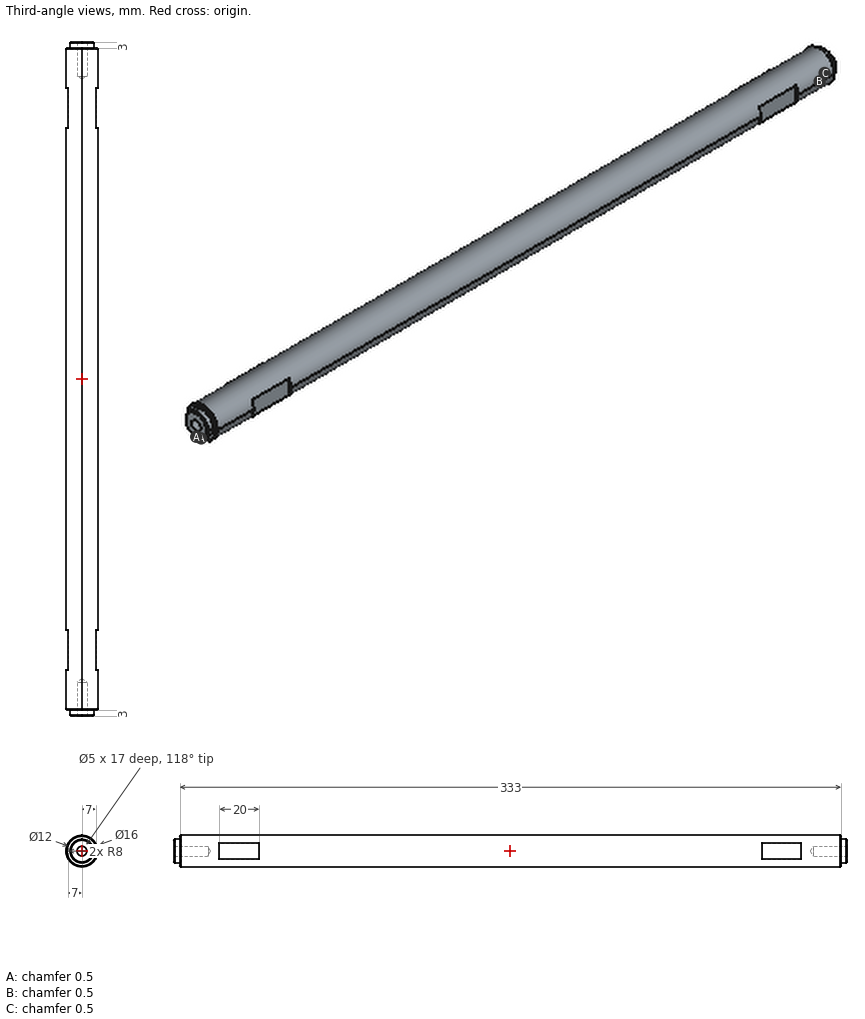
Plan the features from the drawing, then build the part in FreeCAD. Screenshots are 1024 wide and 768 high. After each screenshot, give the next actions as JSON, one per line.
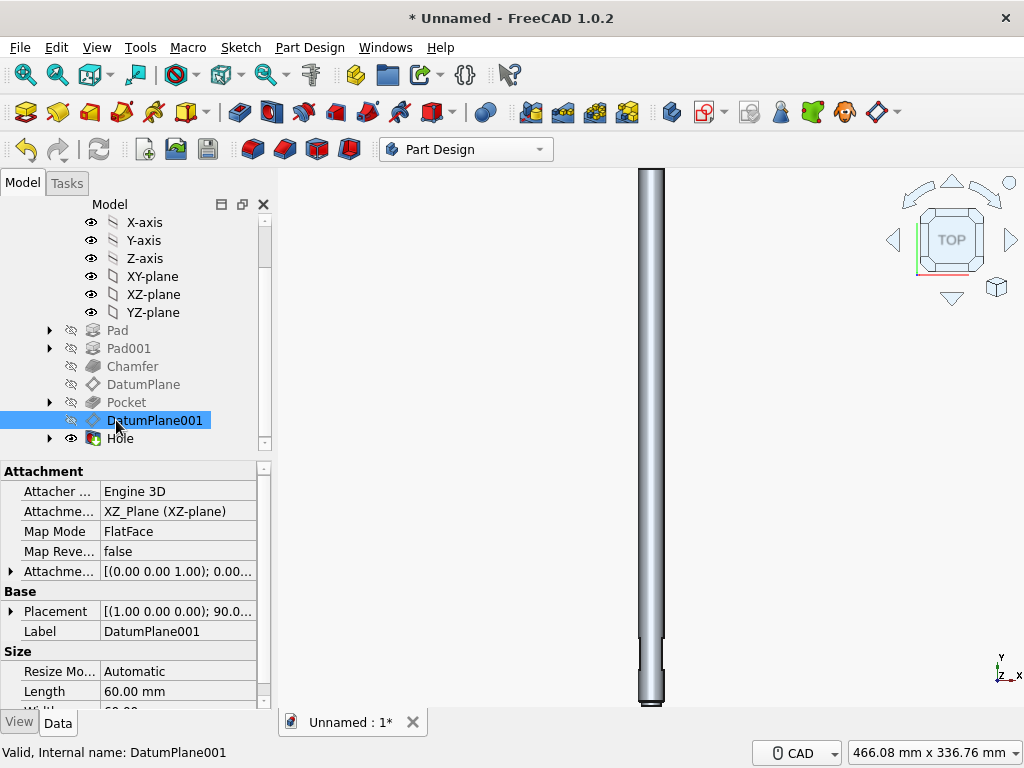
{"action": "key", "text": "0"}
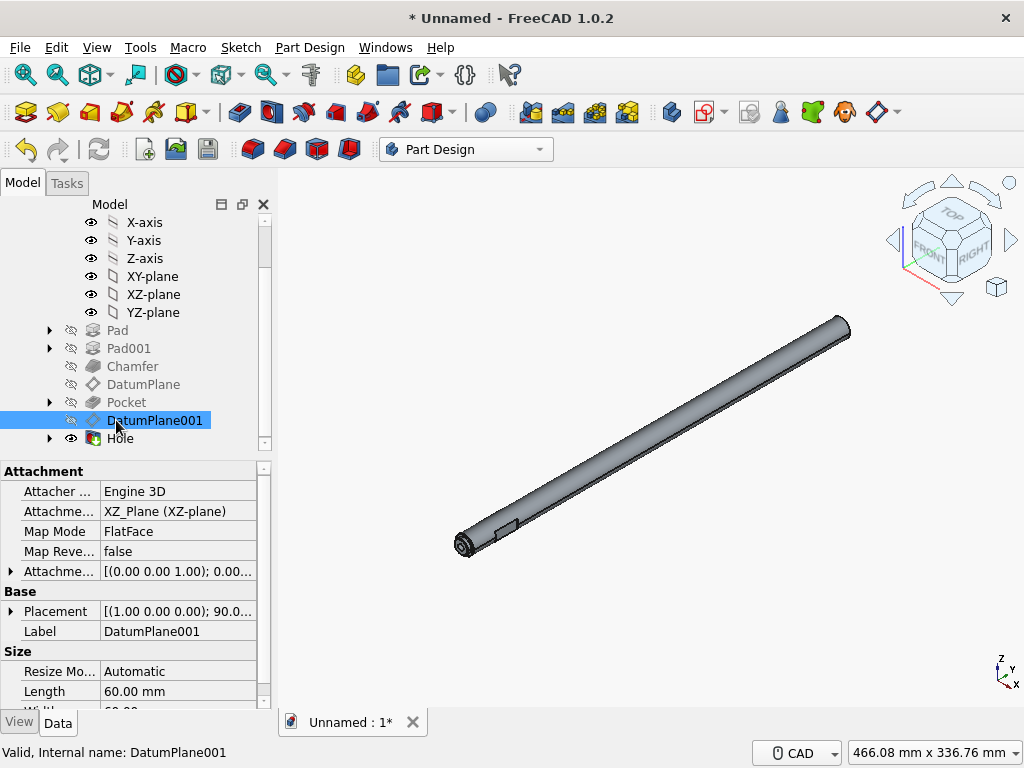
{"action": "left_click", "coordinate": [838, 315]}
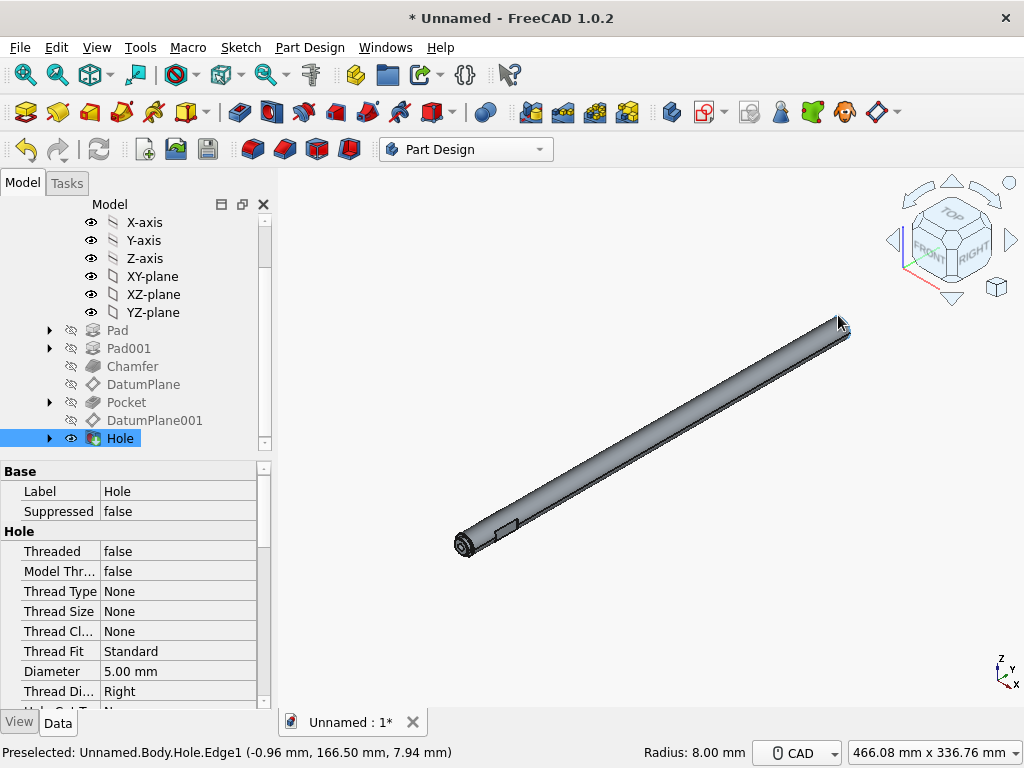
{"action": "left_click", "coordinate": [286, 150]}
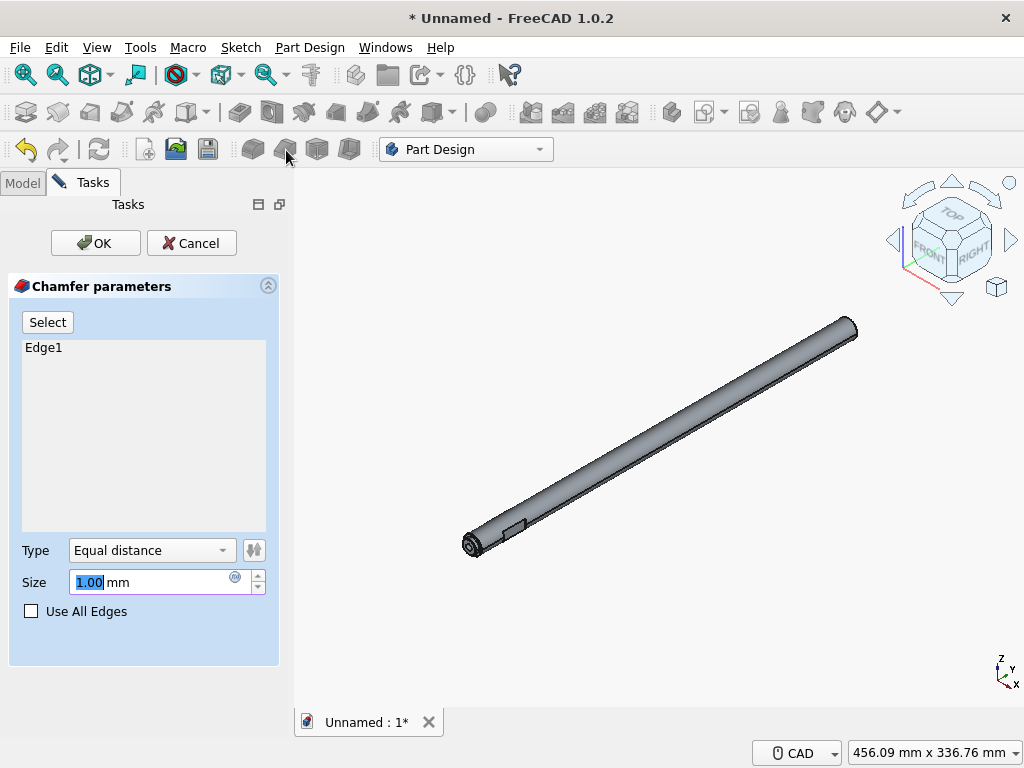
{"action": "type", "text": "0.5"}
{"action": "key", "text": "Tab"}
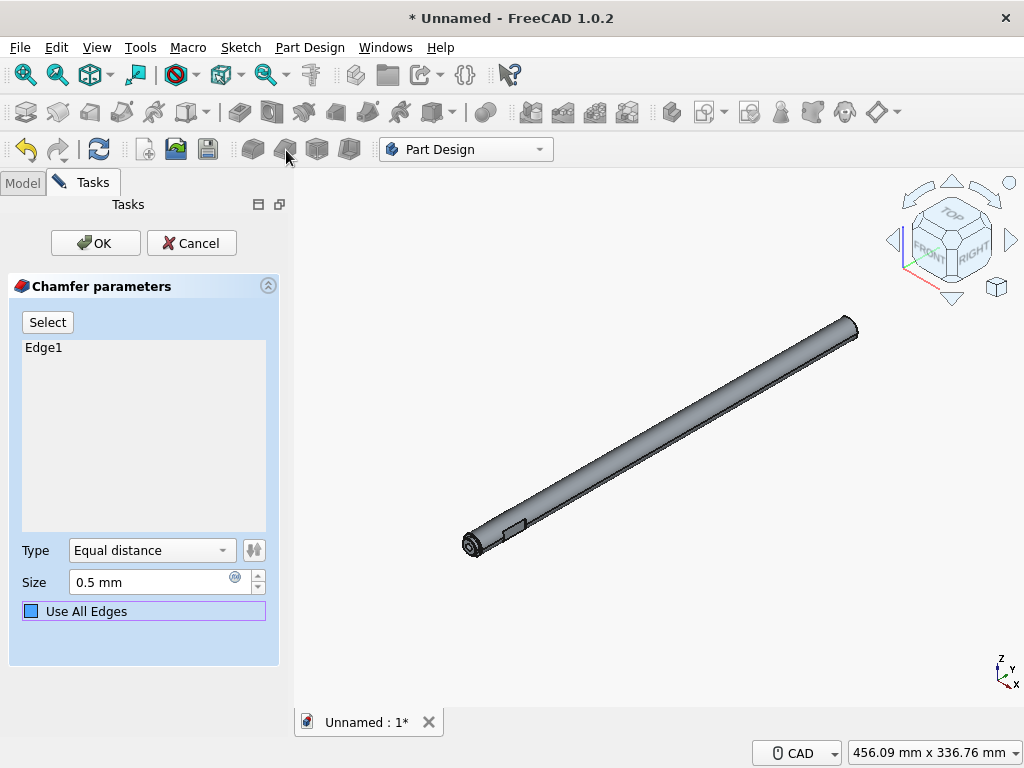
{"action": "left_click", "coordinate": [96, 243]}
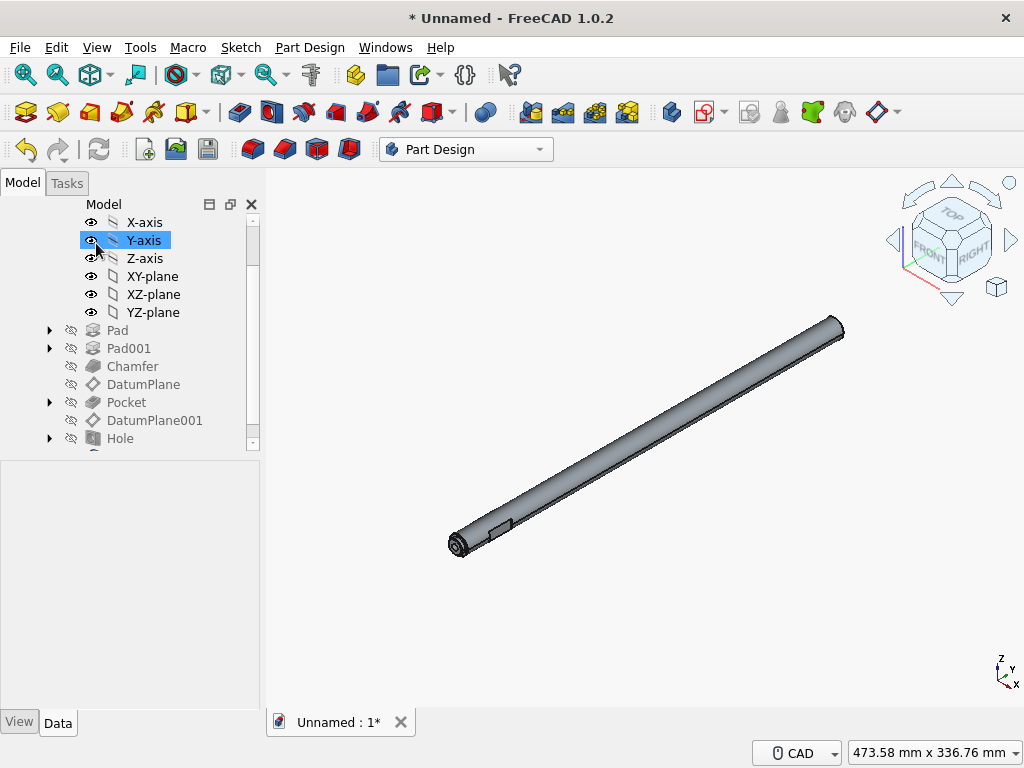
{"action": "scroll", "coordinate": [160, 326], "scroll_direction": "down", "scroll_amount": 3}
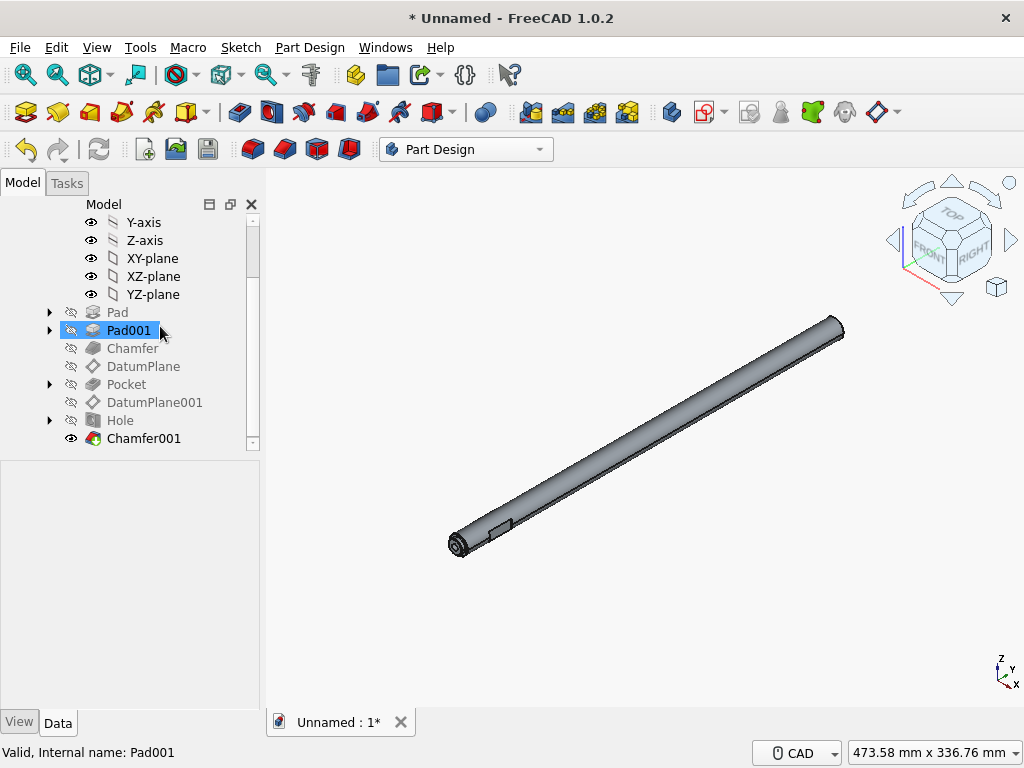
{"action": "scroll", "coordinate": [160, 326], "scroll_direction": "up", "scroll_amount": 15}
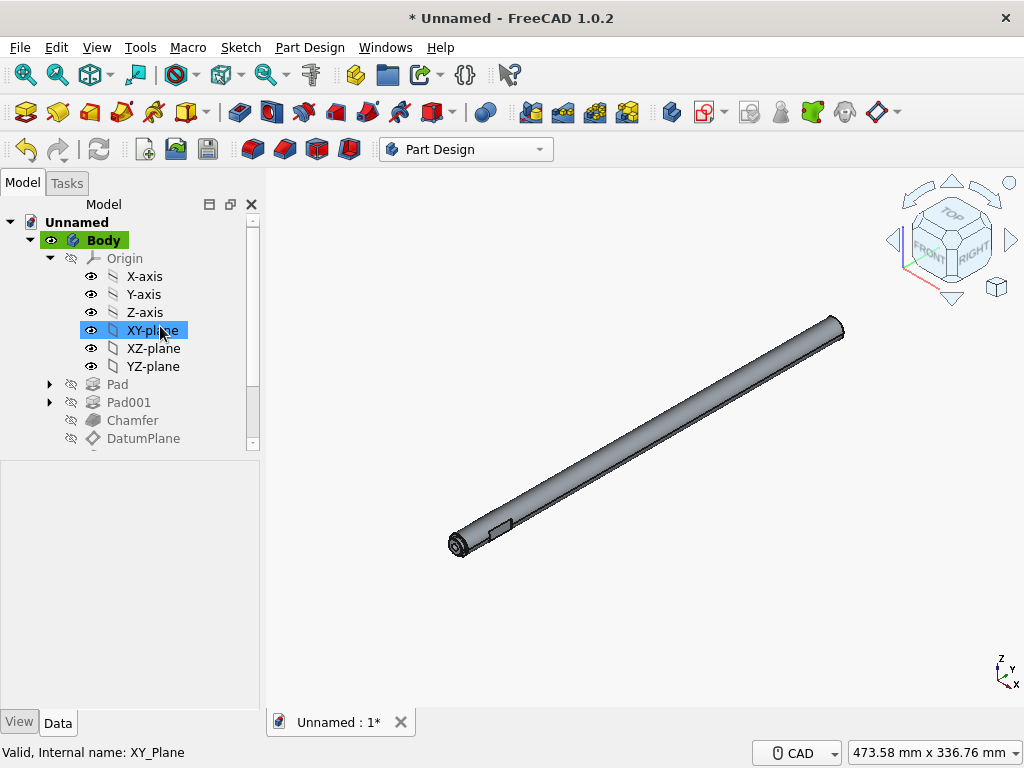
{"action": "left_click", "coordinate": [136, 348]}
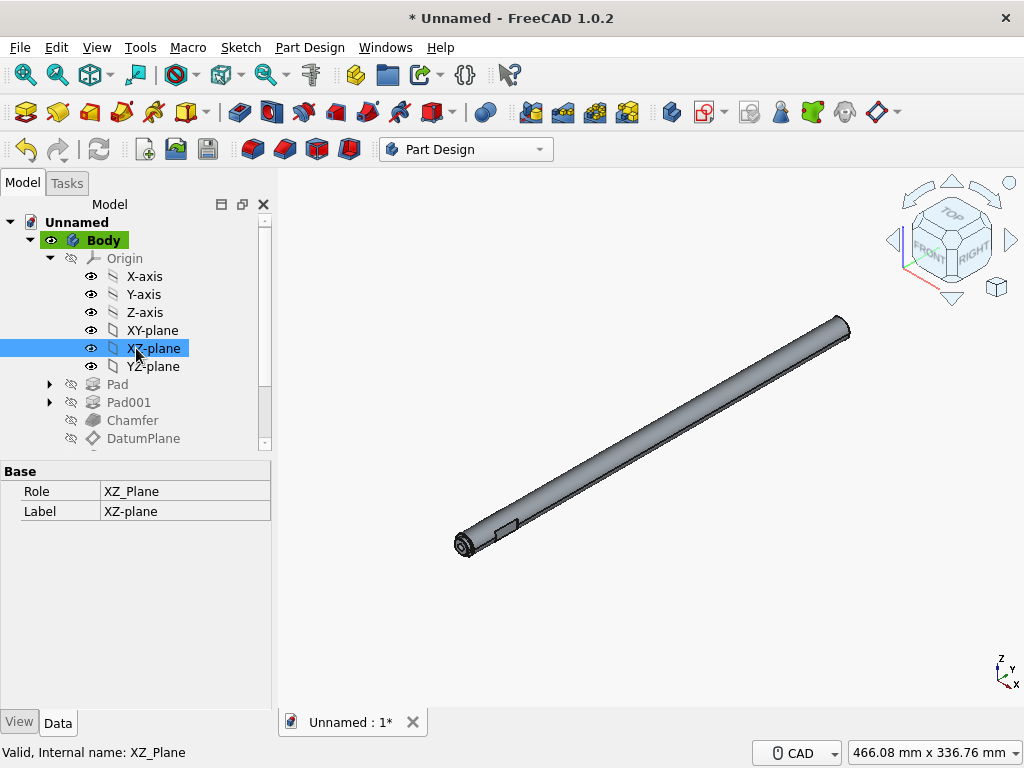
{"action": "left_click", "coordinate": [878, 112]}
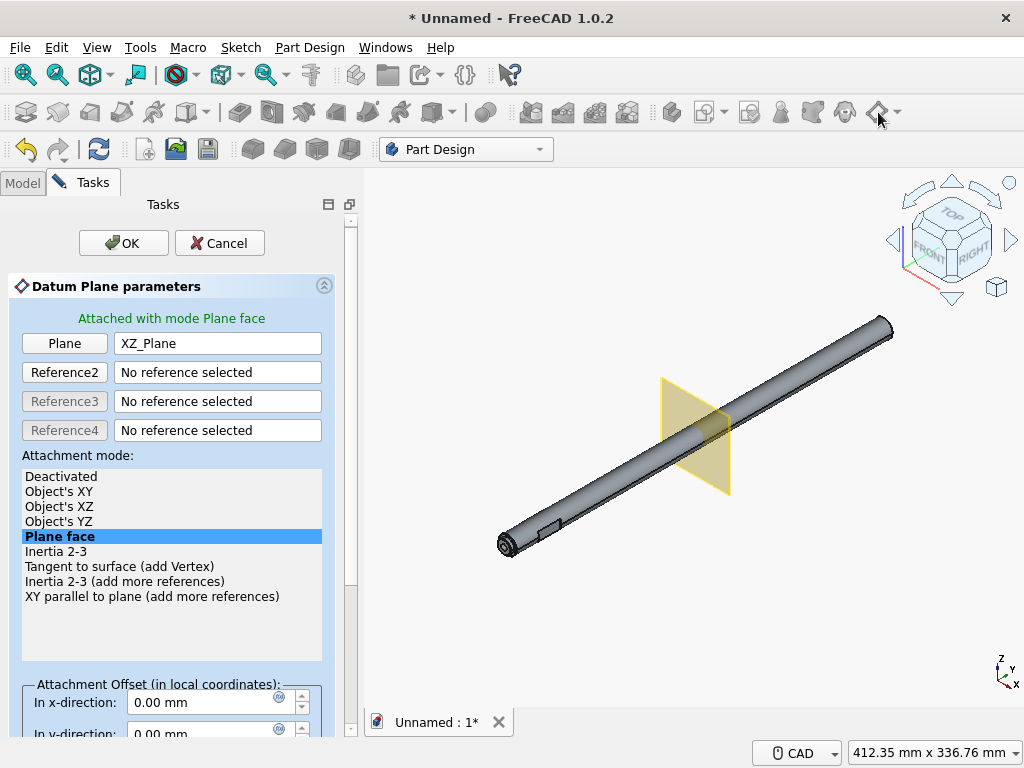
{"action": "scroll", "coordinate": [351, 475], "scroll_direction": "down", "scroll_amount": 2}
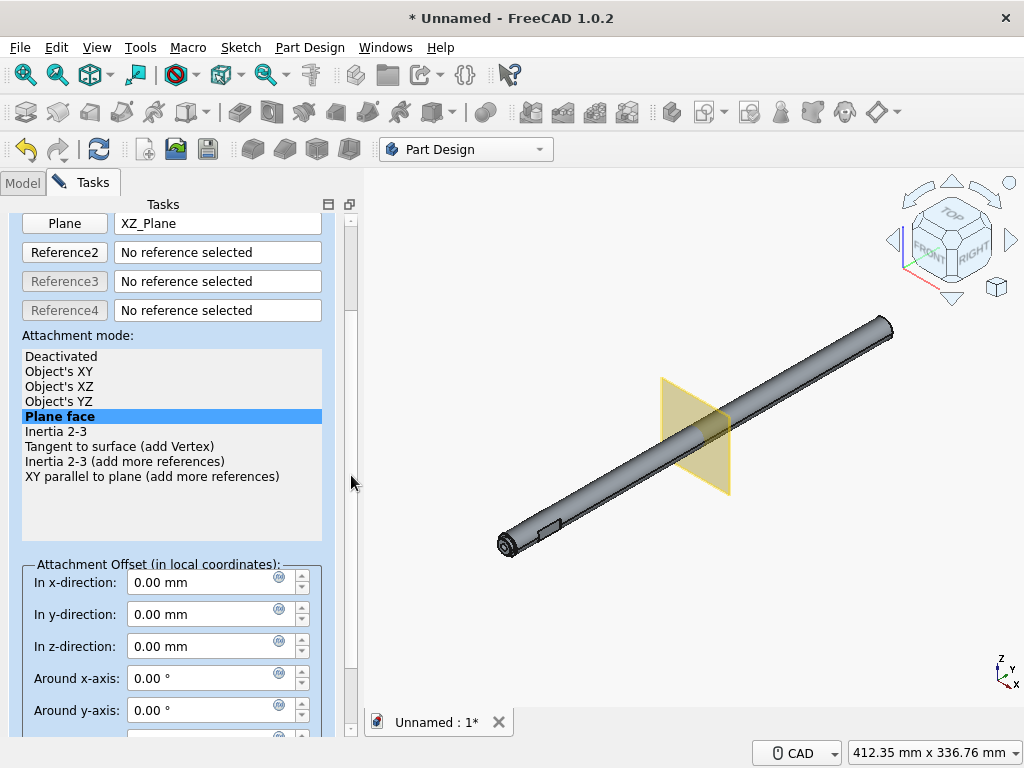
{"action": "triple_click", "coordinate": [210, 646]}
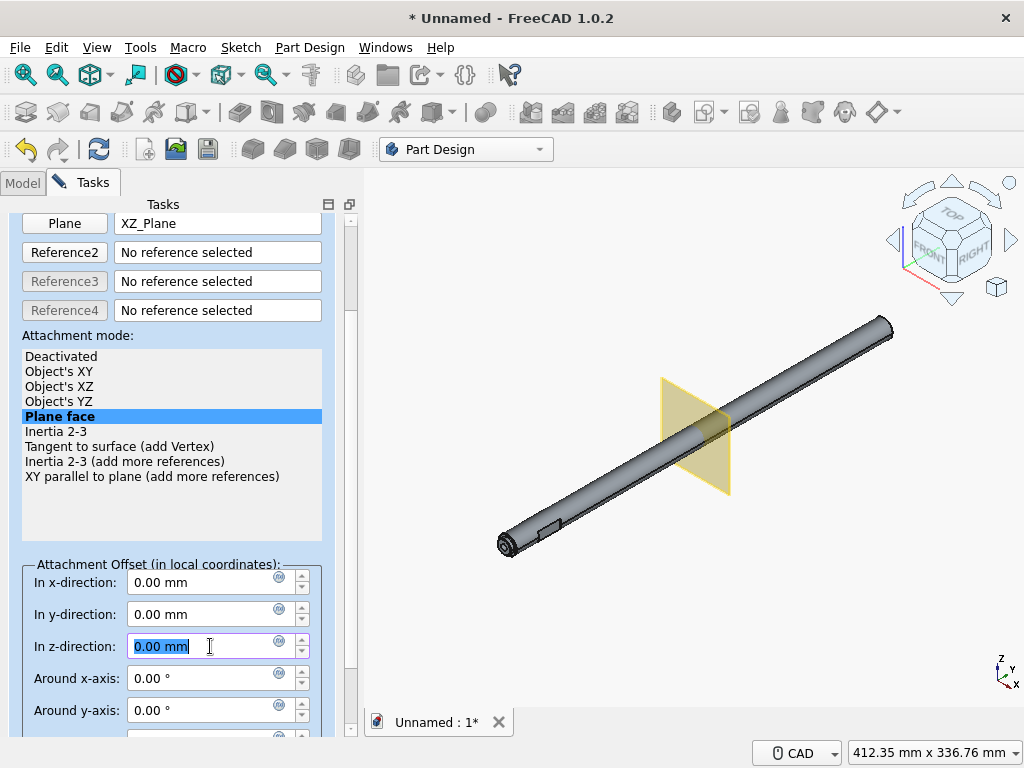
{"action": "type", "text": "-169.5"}
{"action": "key", "text": "Tab"}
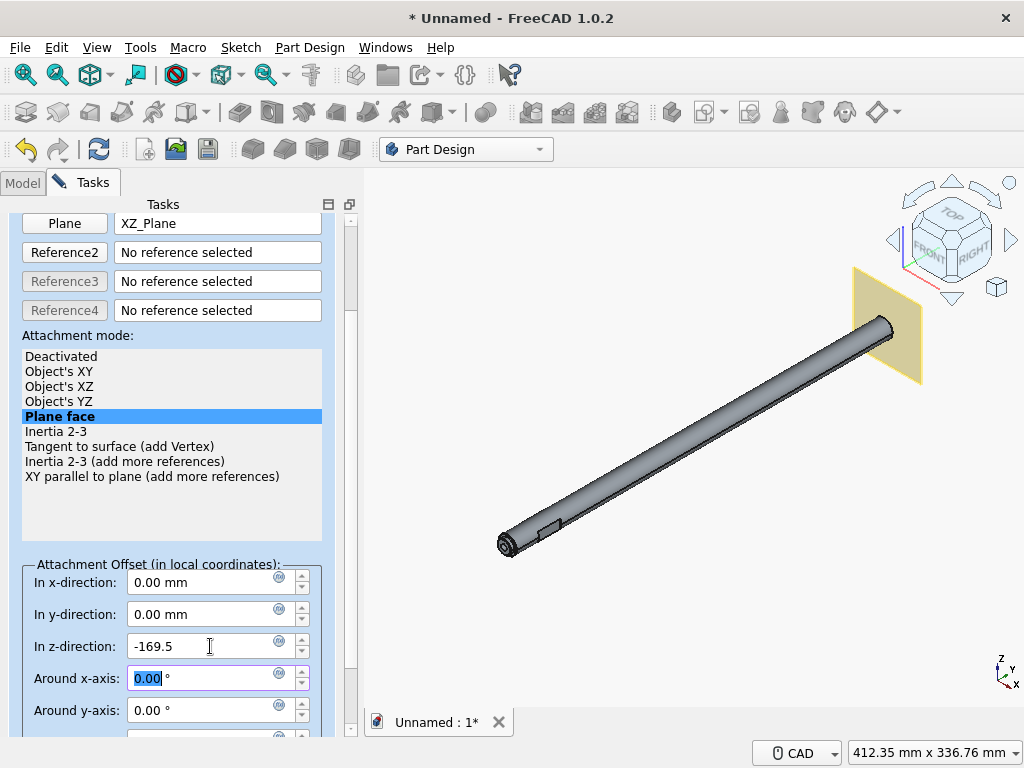
{"action": "scroll", "coordinate": [351, 475], "scroll_direction": "up", "scroll_amount": 3}